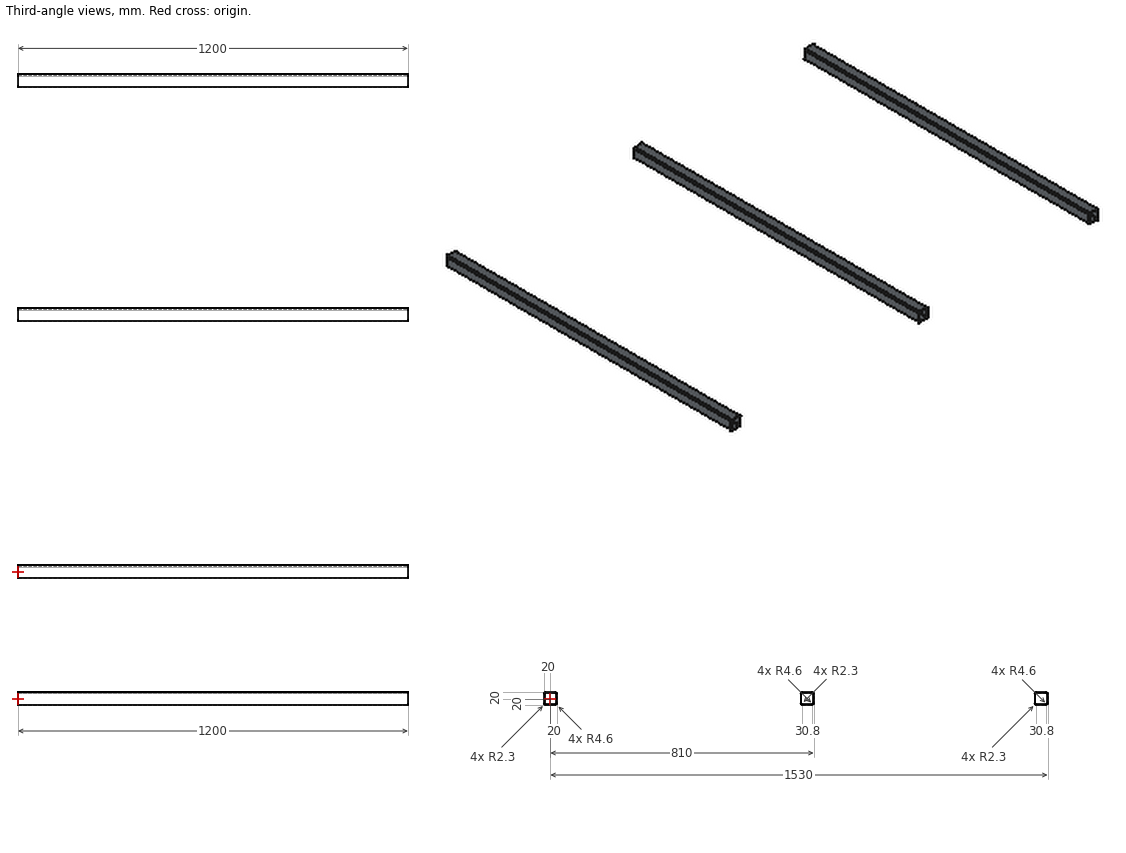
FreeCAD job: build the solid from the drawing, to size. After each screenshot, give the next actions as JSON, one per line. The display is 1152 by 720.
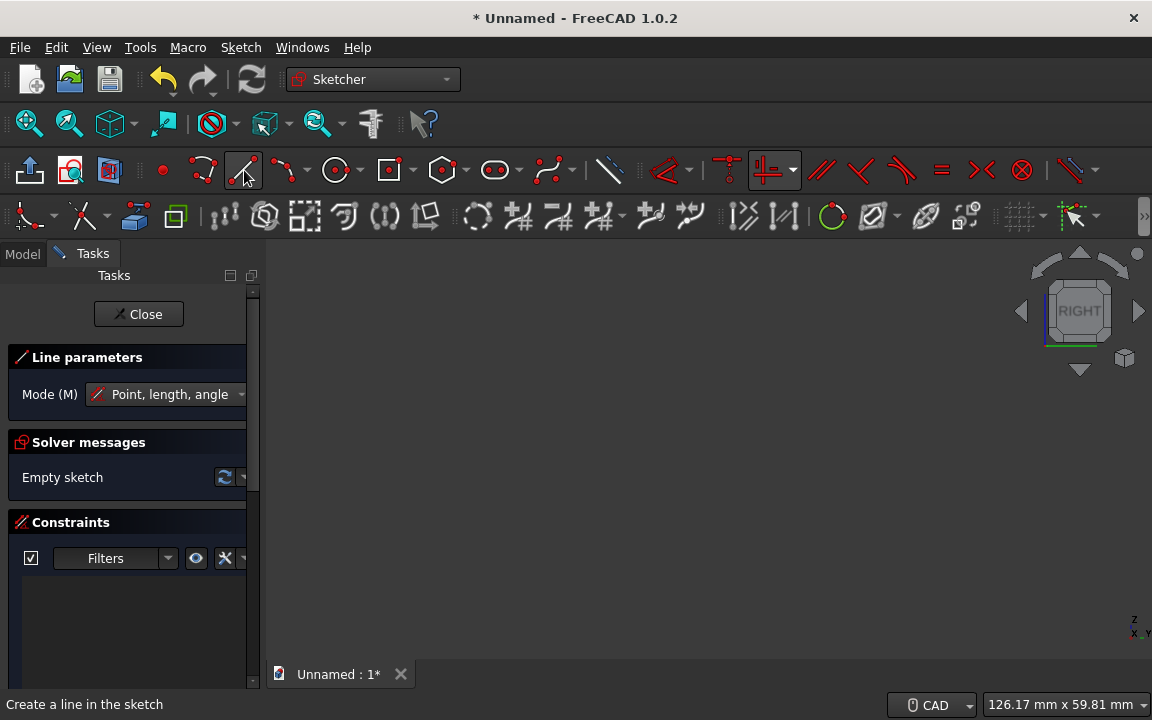
{"action": "left_click", "coordinate": [531, 588]}
{"action": "left_click", "coordinate": [747, 588]}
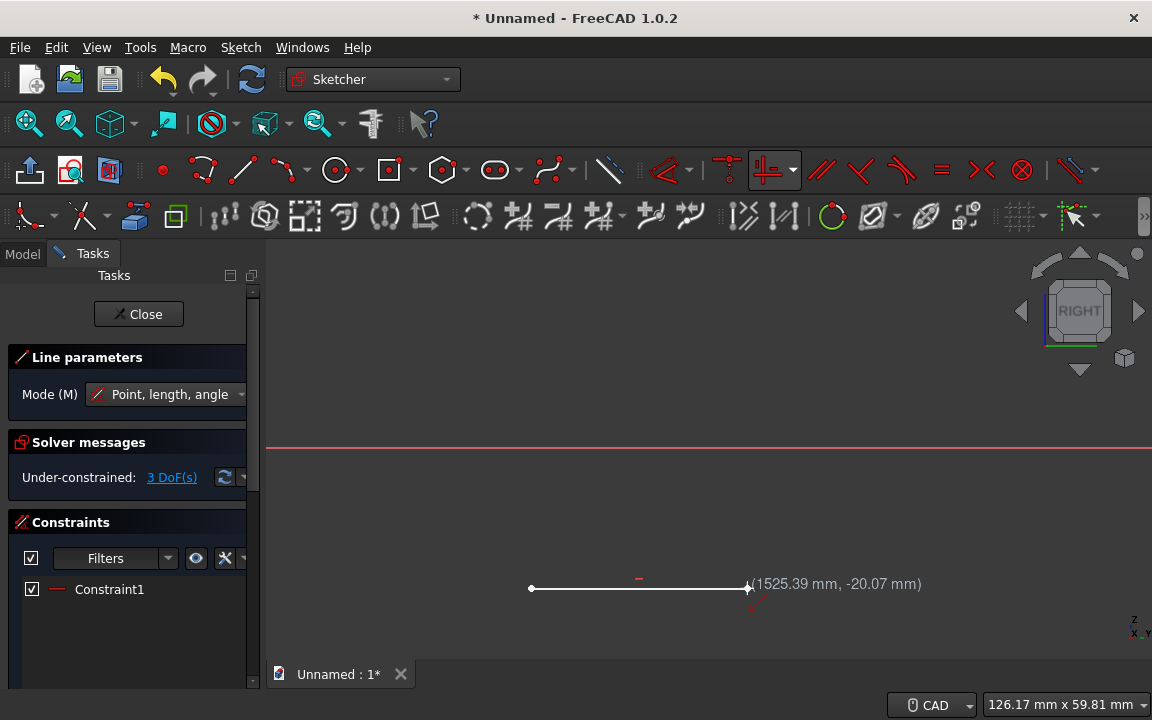
{"action": "left_click", "coordinate": [779, 556]}
{"action": "left_click", "coordinate": [779, 340]}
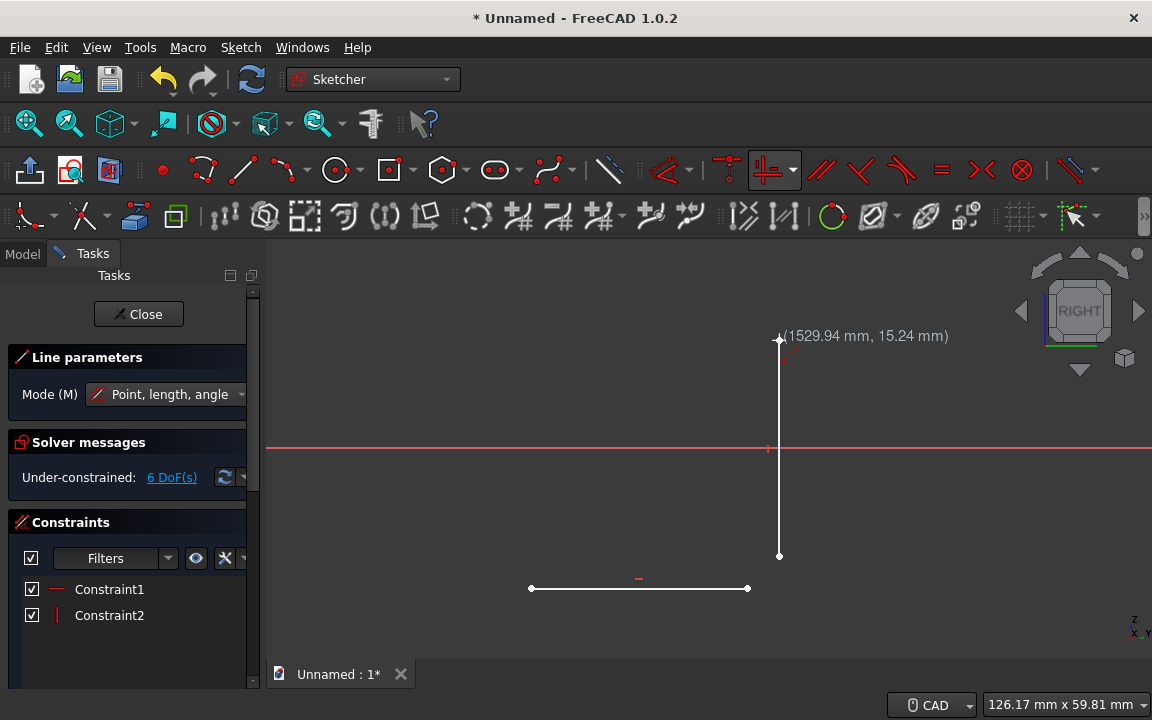
{"action": "left_click", "coordinate": [747, 308]}
{"action": "left_click", "coordinate": [531, 308]}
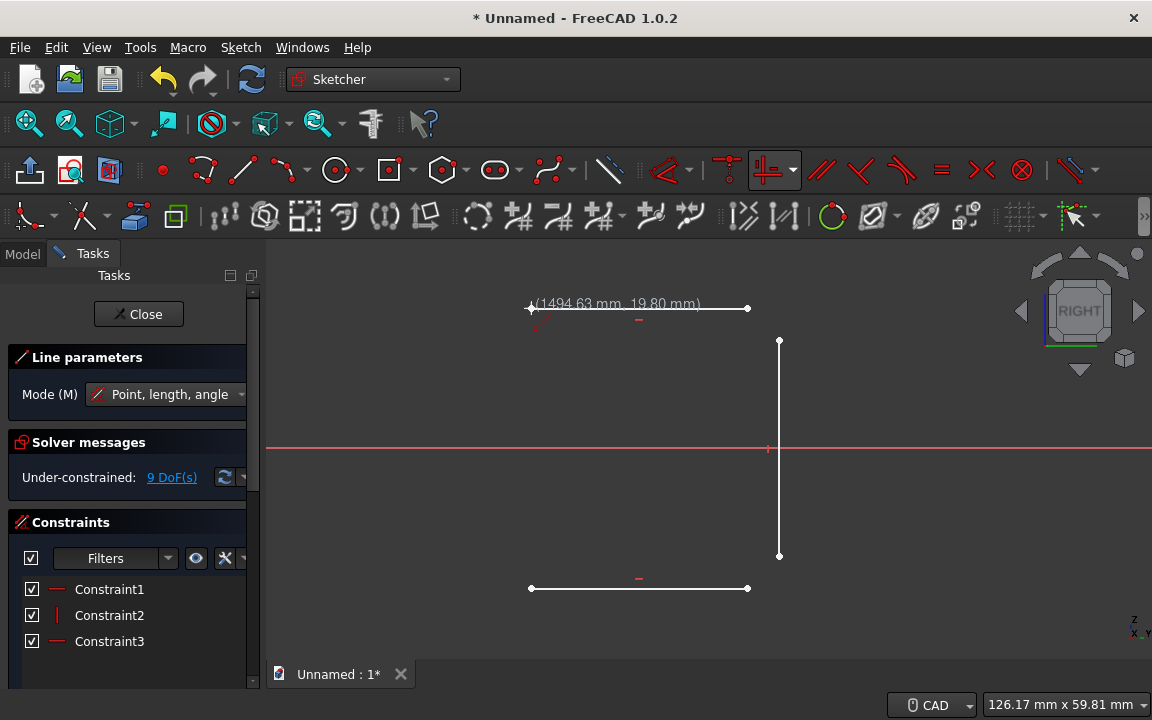
{"action": "left_click", "coordinate": [499, 340]}
{"action": "left_click", "coordinate": [499, 556]}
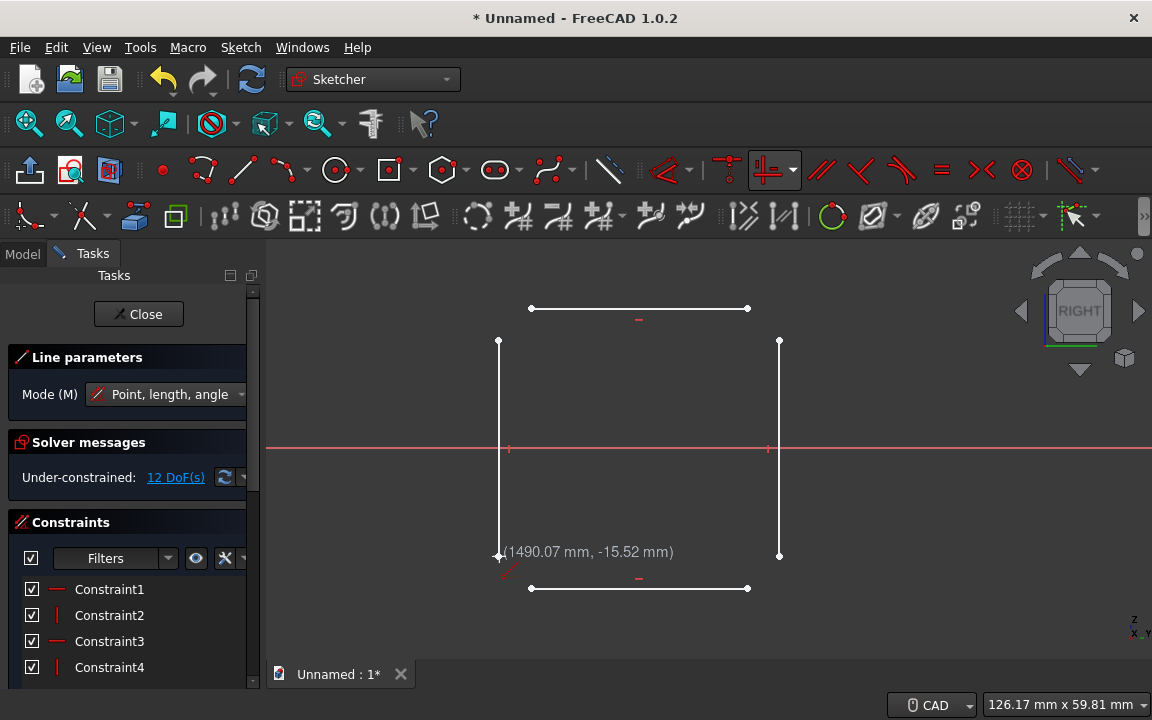
{"action": "key", "text": "g 3 a"}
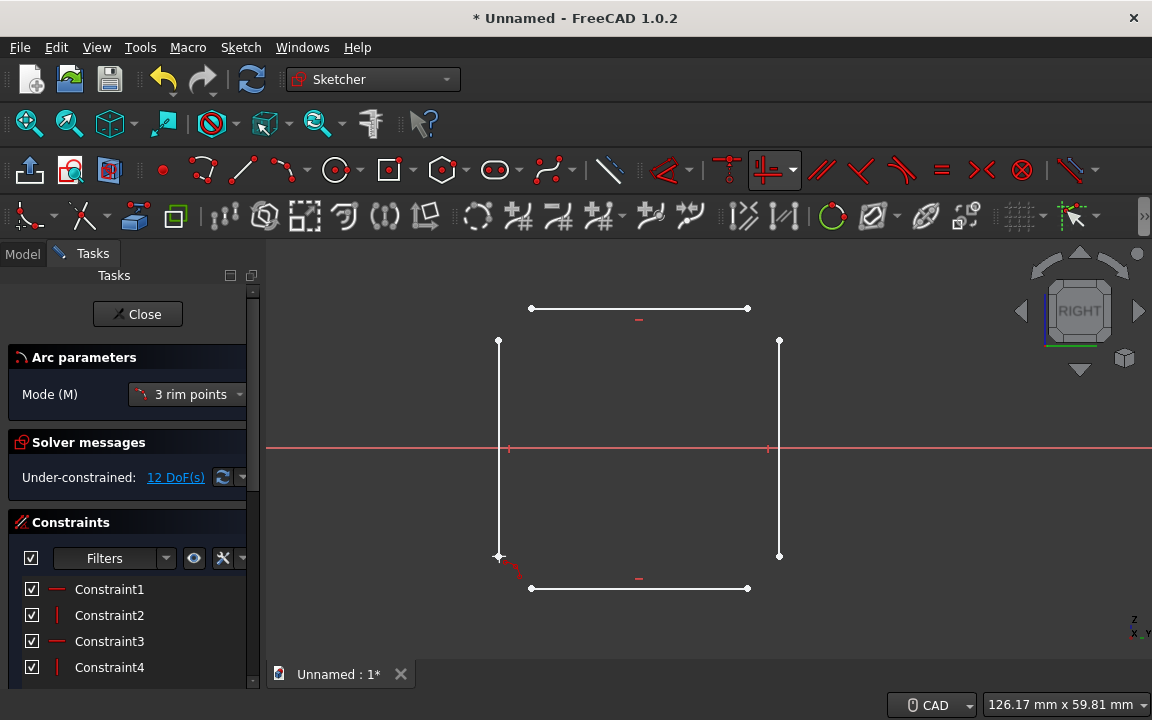
{"action": "left_click", "coordinate": [747, 589]}
{"action": "left_click", "coordinate": [779, 557]}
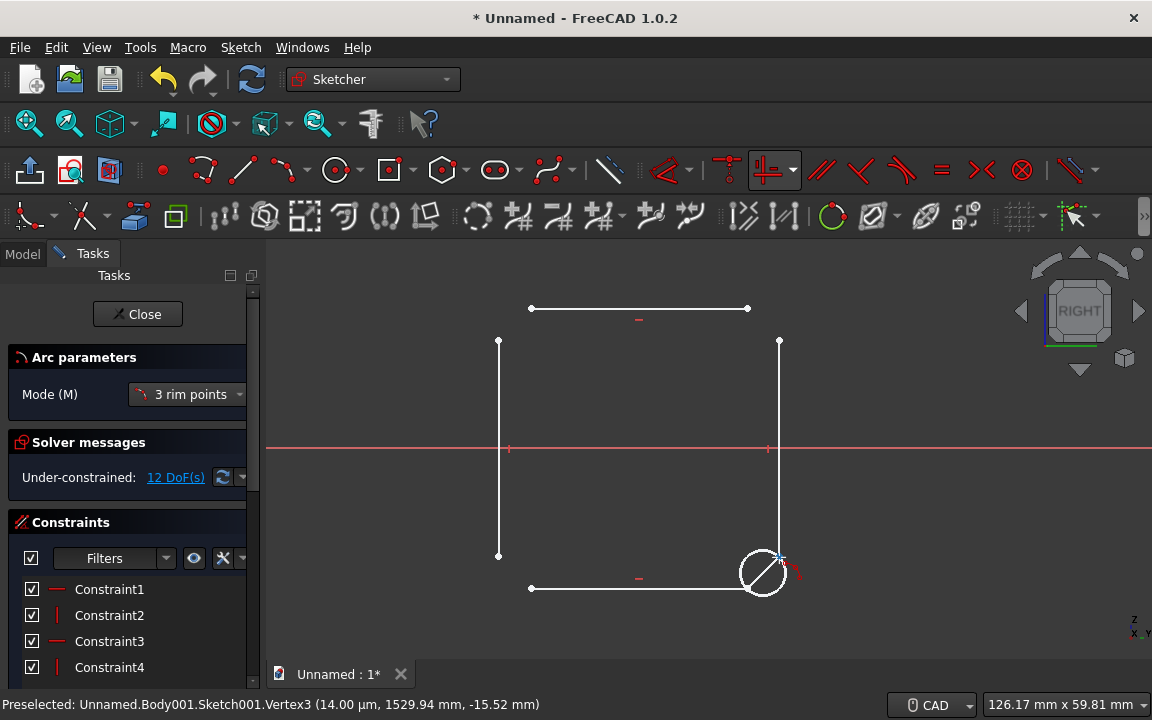
{"action": "scroll", "coordinate": [770, 579], "scroll_direction": "up", "scroll_amount": 3}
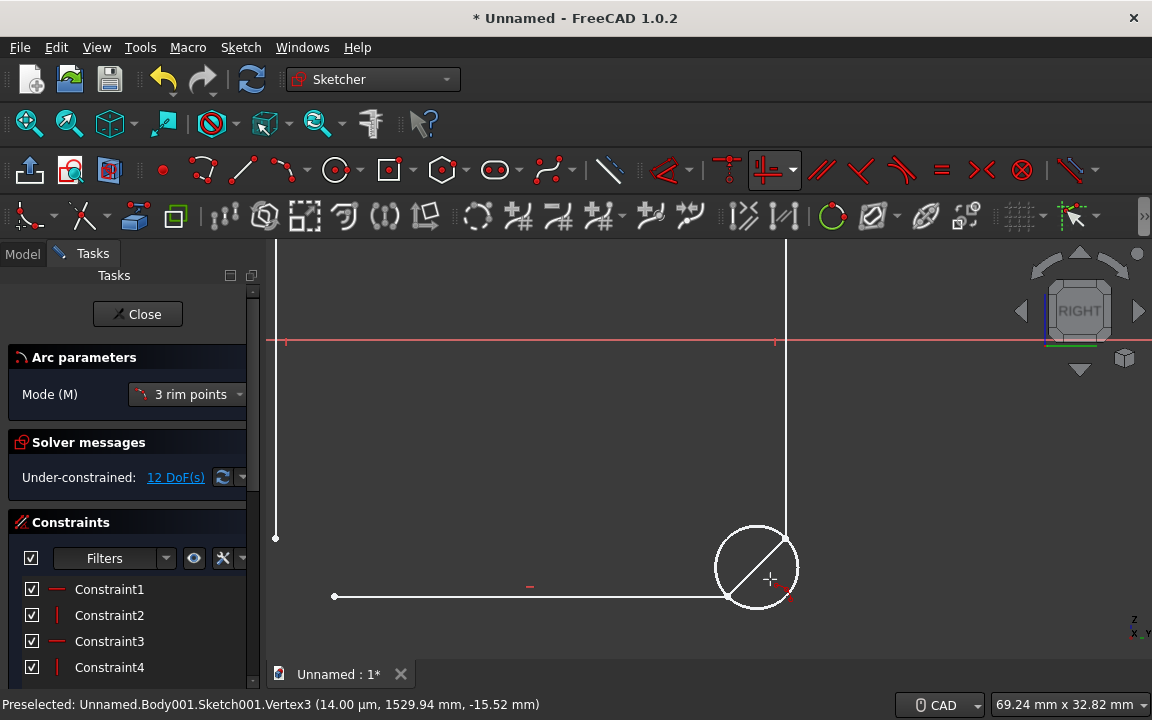
{"action": "left_click", "coordinate": [769, 578]}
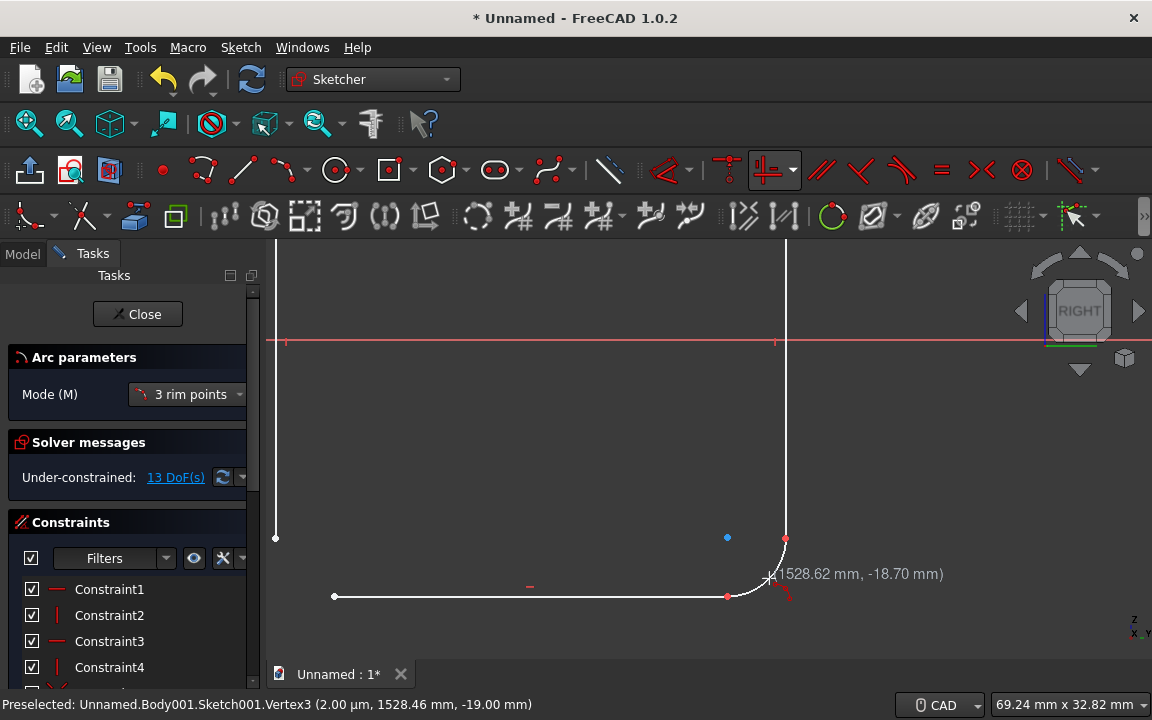
{"action": "scroll", "coordinate": [774, 582], "scroll_direction": "down", "scroll_amount": 3}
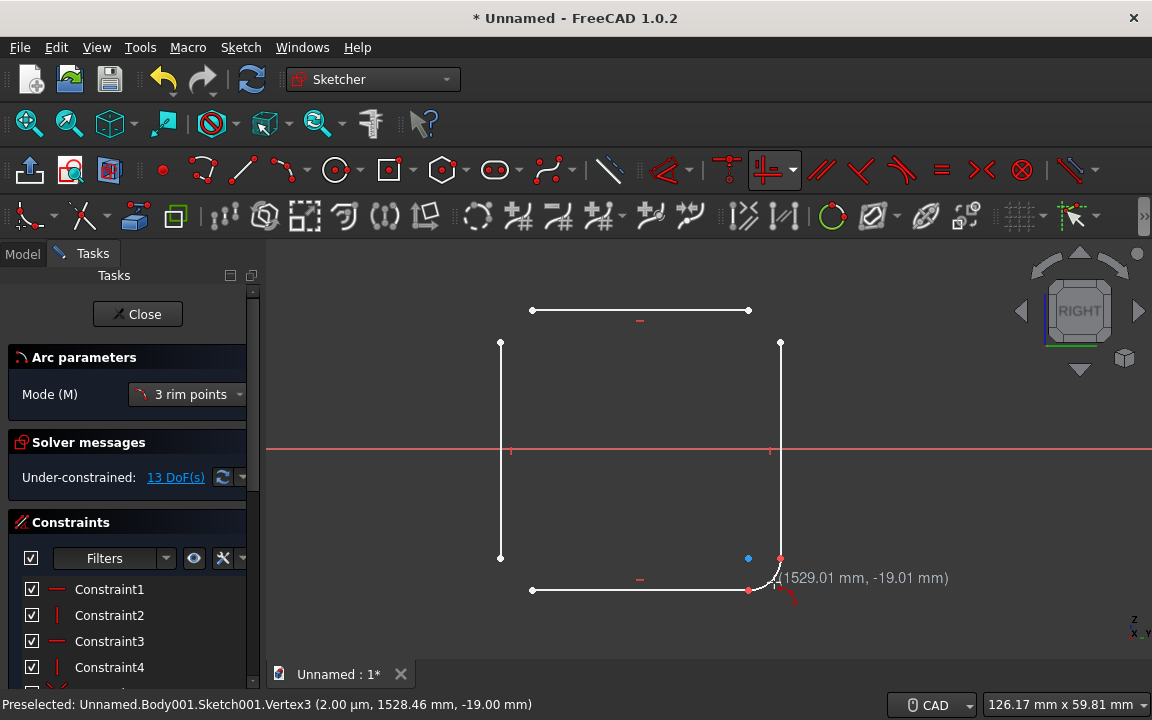
{"action": "left_click", "coordinate": [781, 342]}
{"action": "left_click", "coordinate": [749, 310]}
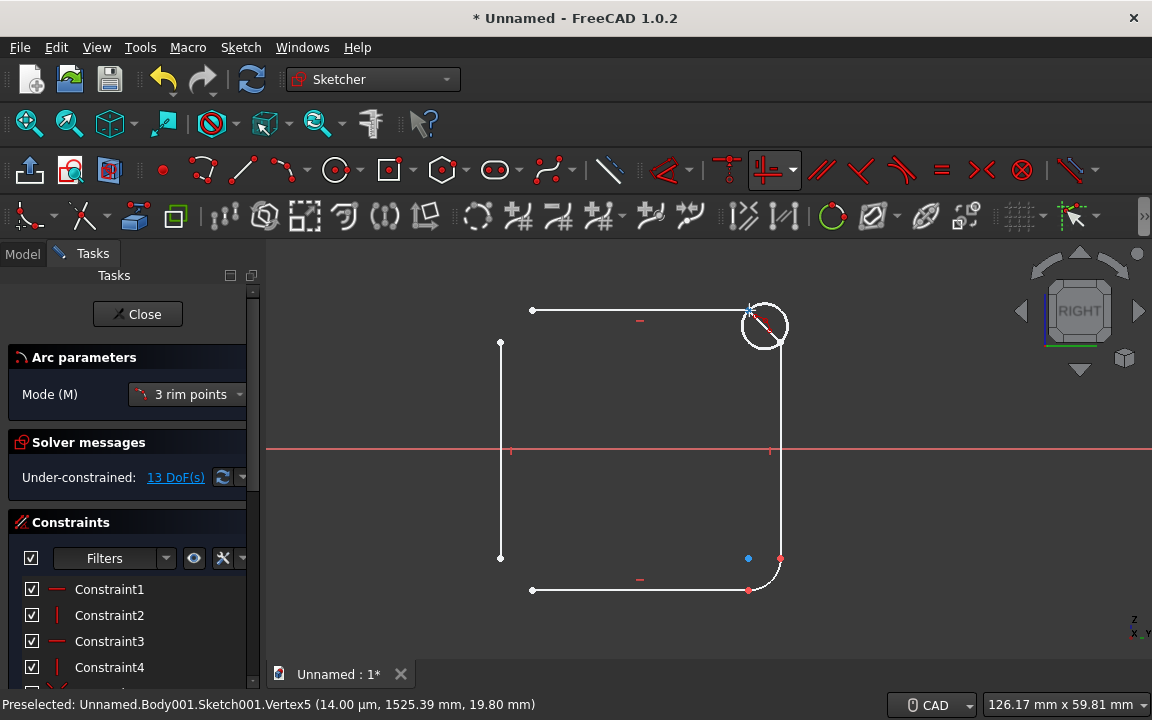
{"action": "scroll", "coordinate": [772, 318], "scroll_direction": "up", "scroll_amount": 3}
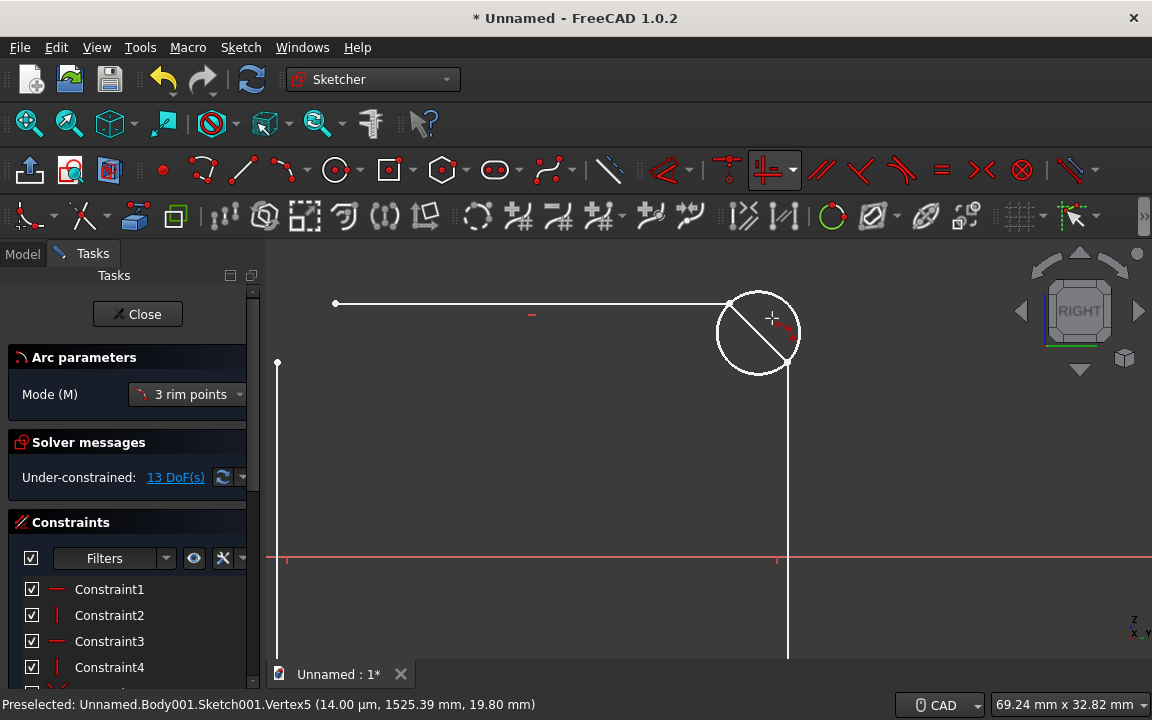
{"action": "left_click", "coordinate": [771, 319]}